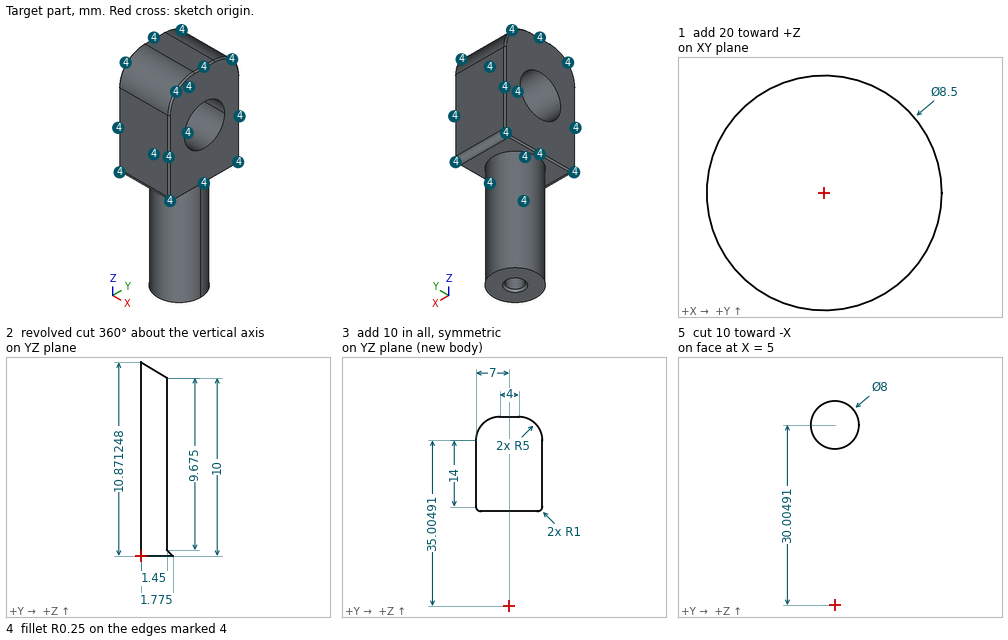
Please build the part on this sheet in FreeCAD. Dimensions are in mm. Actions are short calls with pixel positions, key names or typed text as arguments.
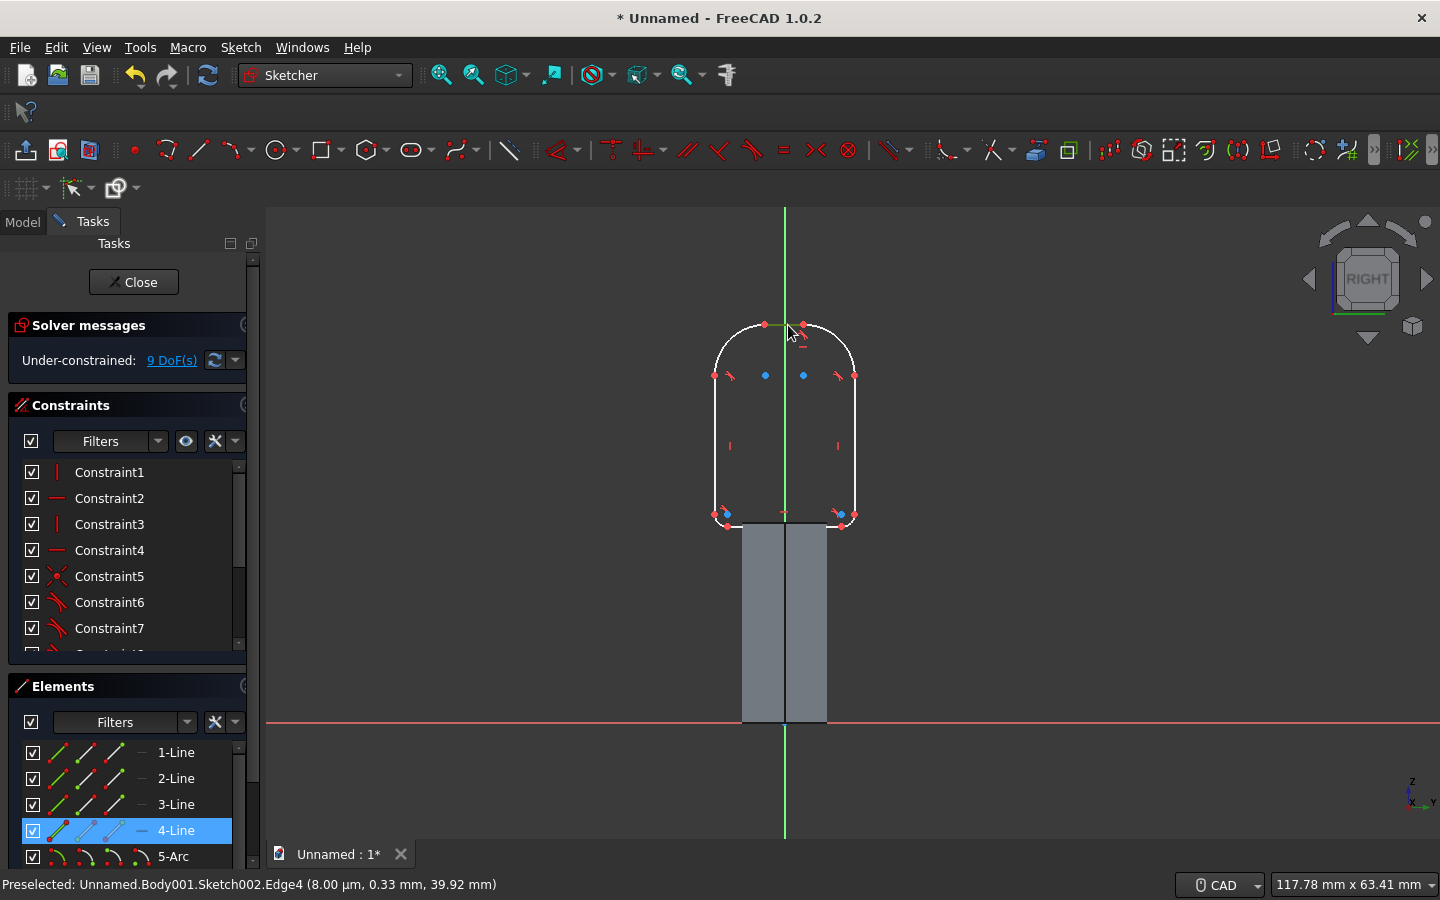
click(742, 331)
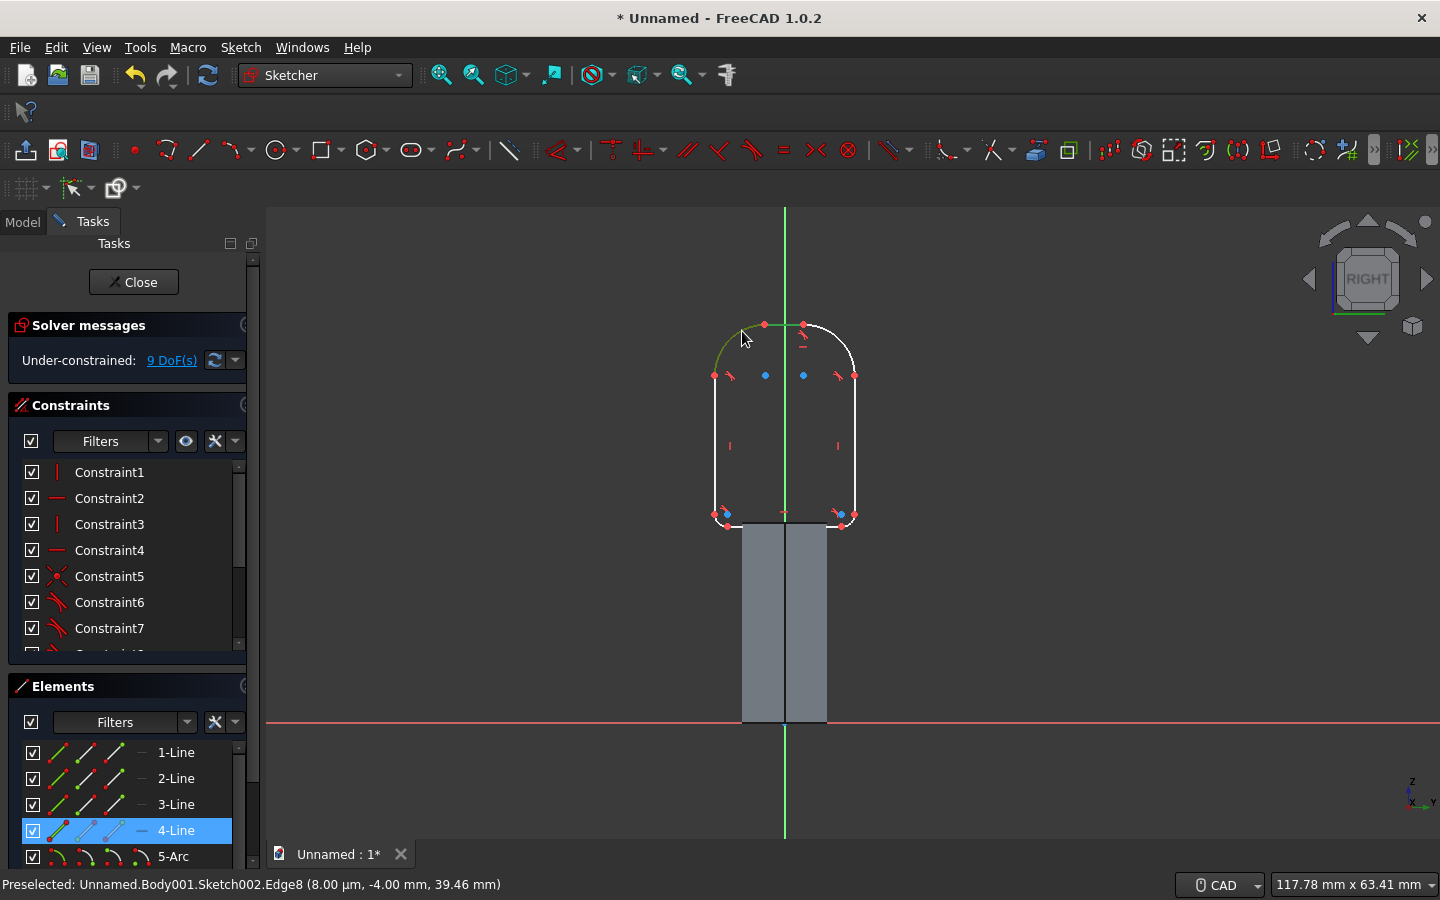
key(t)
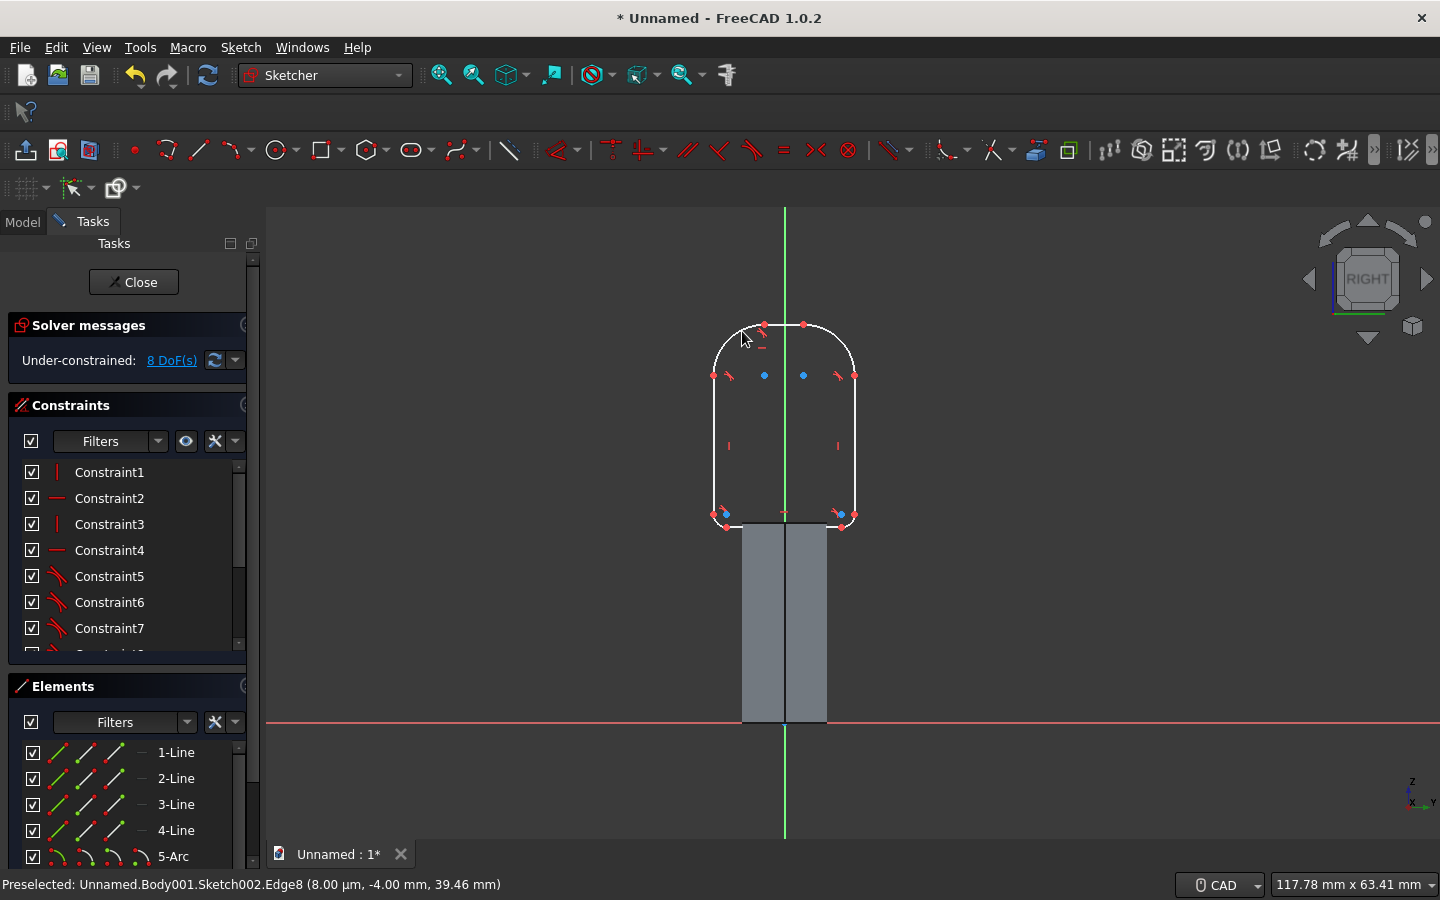
scroll(717, 523, up, 2)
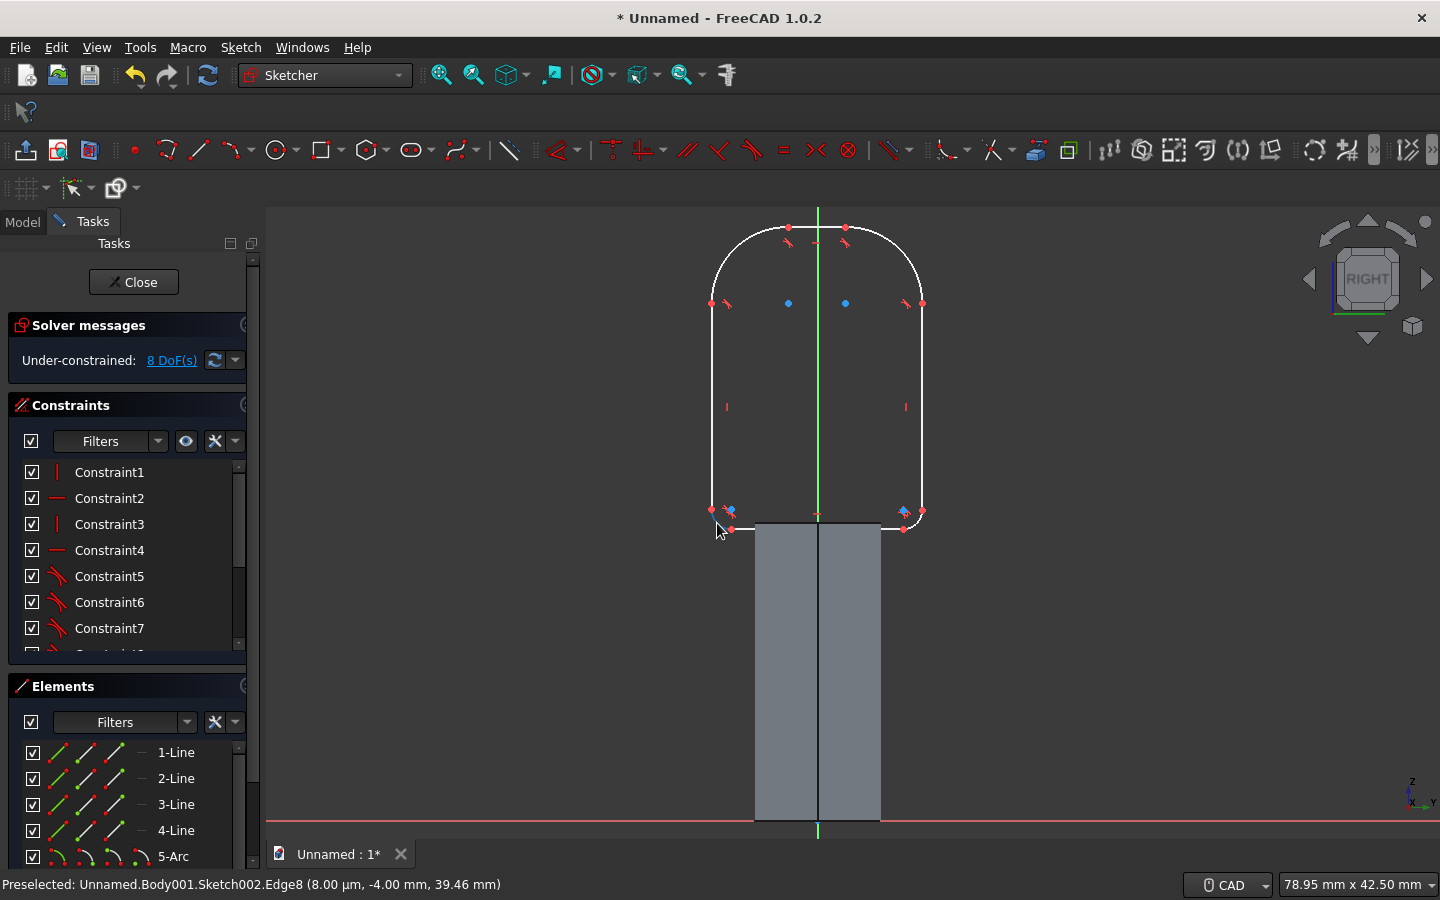
click(717, 523)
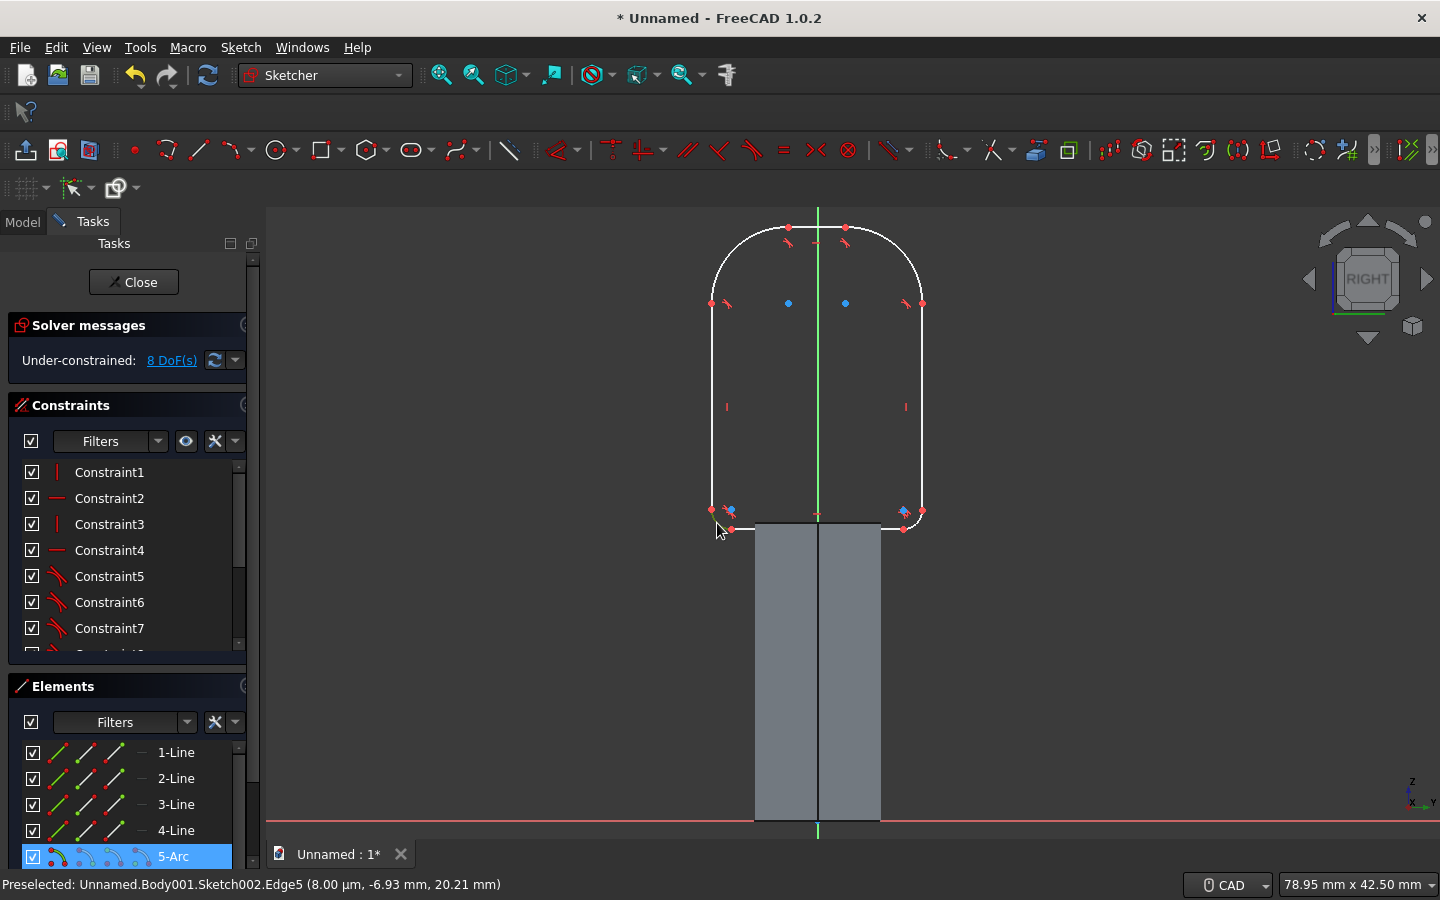
click(917, 524)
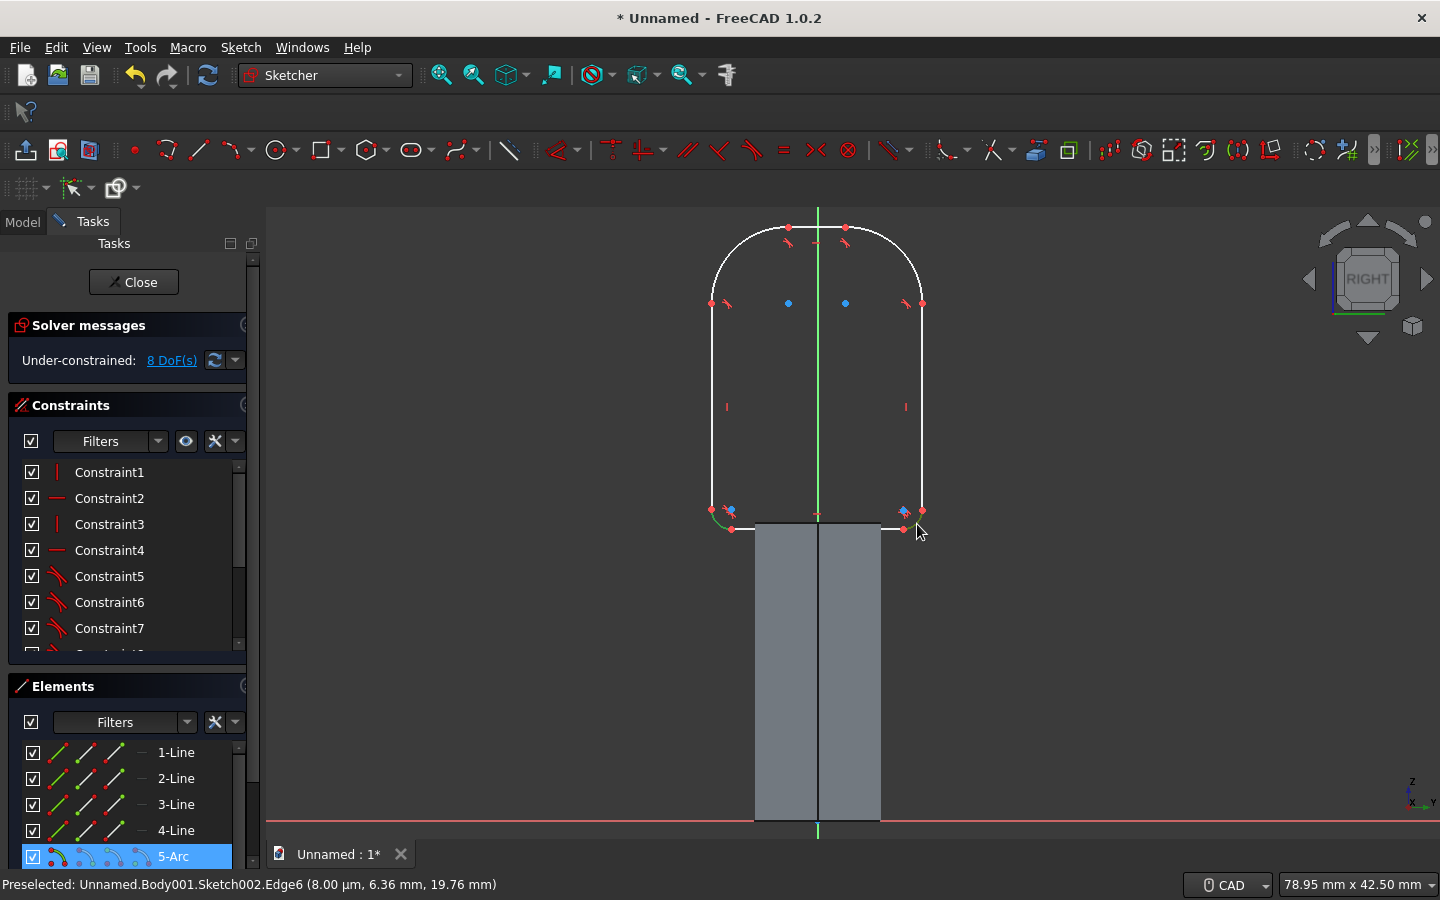
click(784, 150)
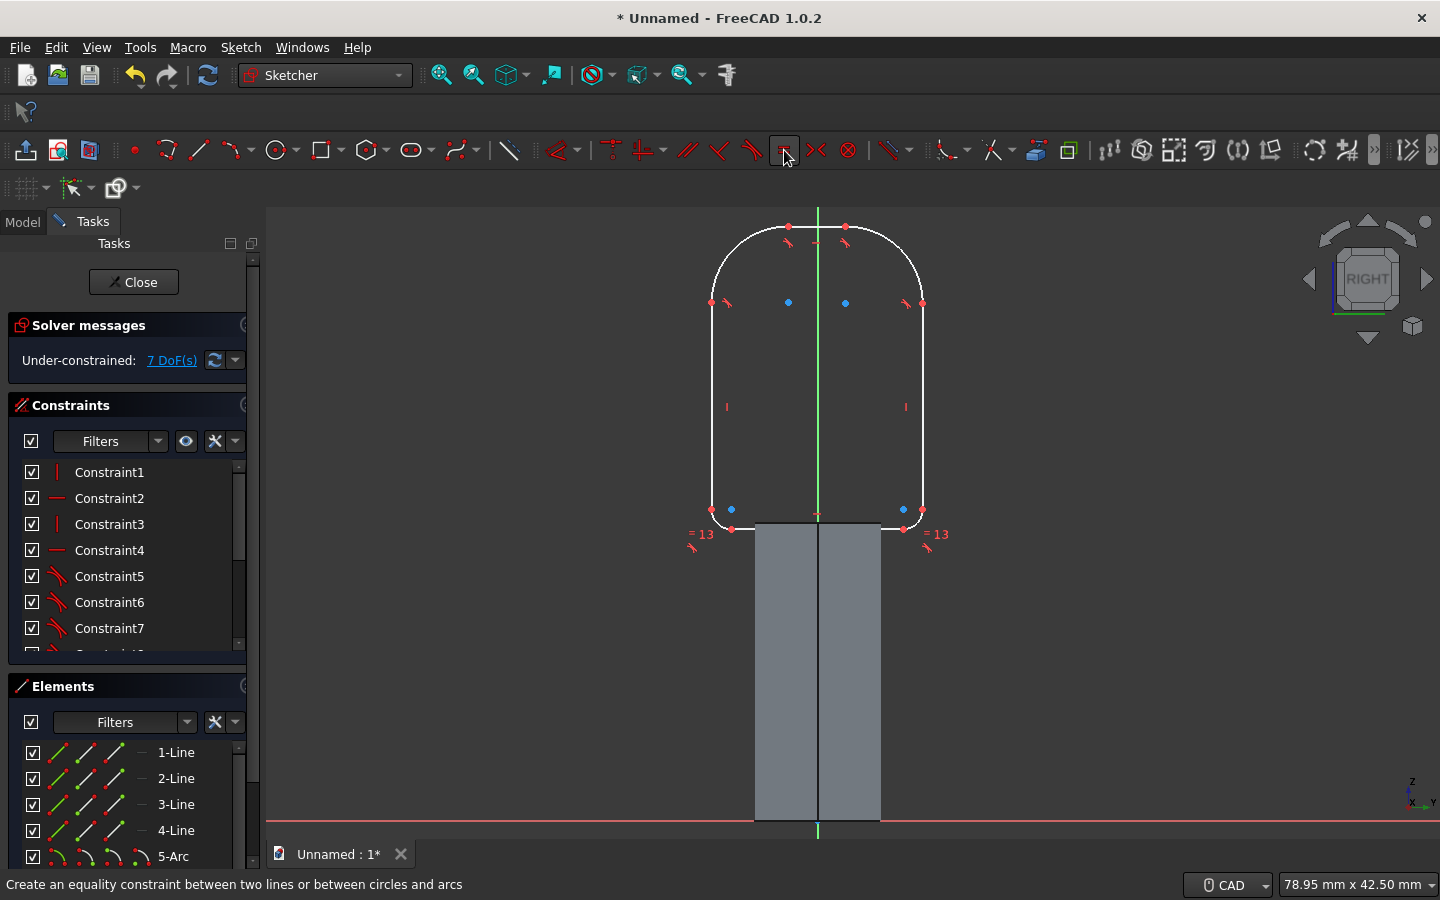
click(914, 269)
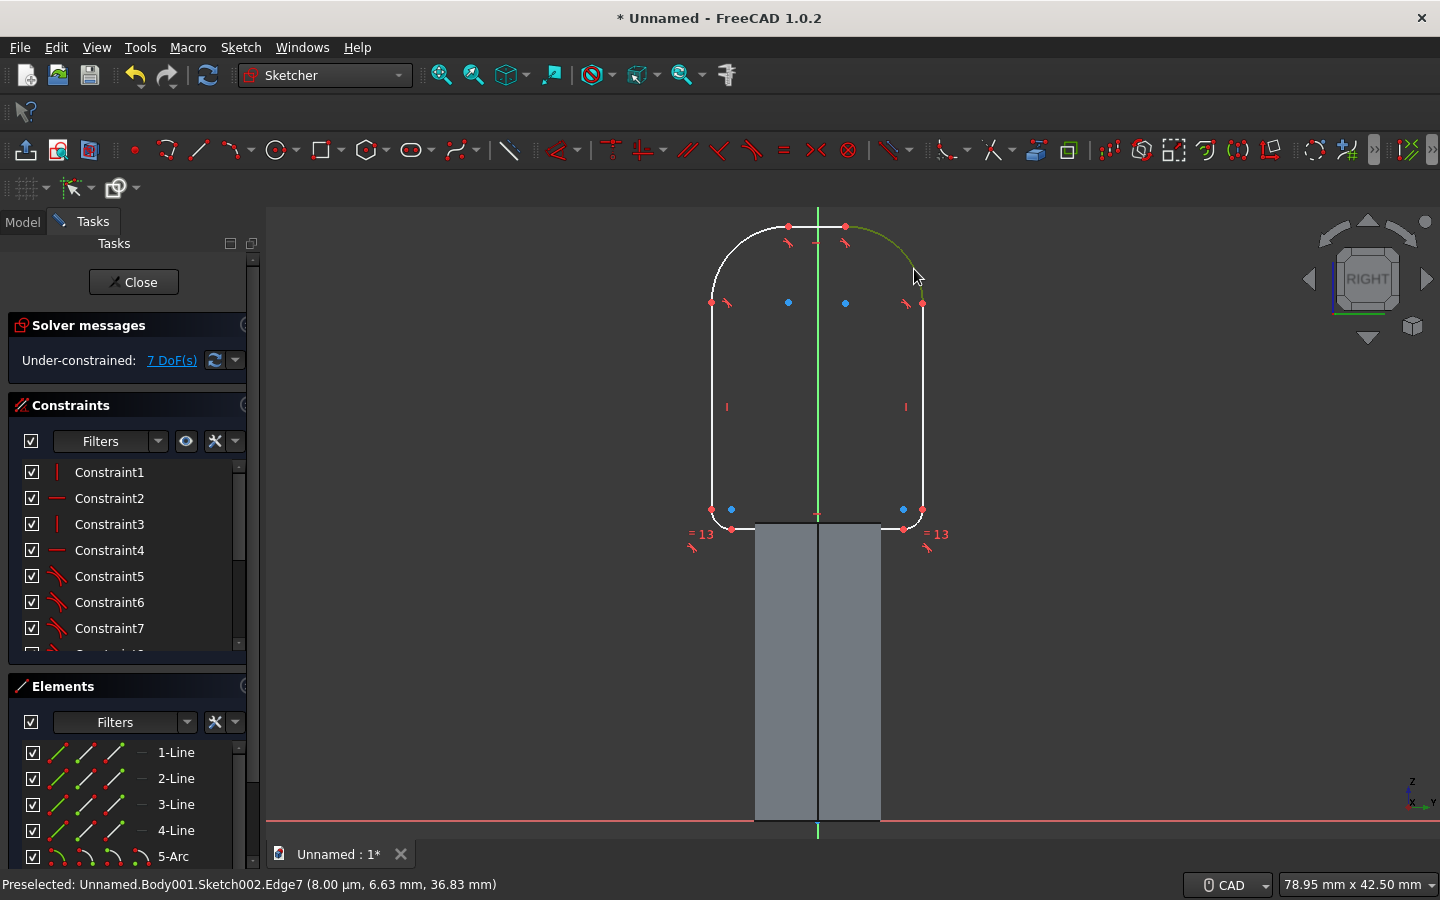
click(720, 268)